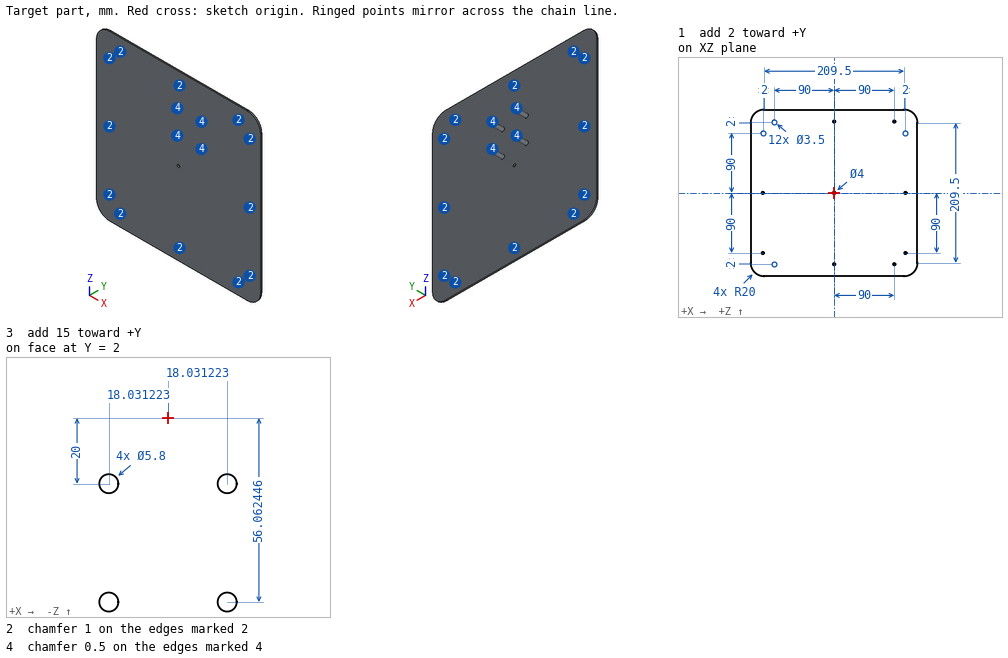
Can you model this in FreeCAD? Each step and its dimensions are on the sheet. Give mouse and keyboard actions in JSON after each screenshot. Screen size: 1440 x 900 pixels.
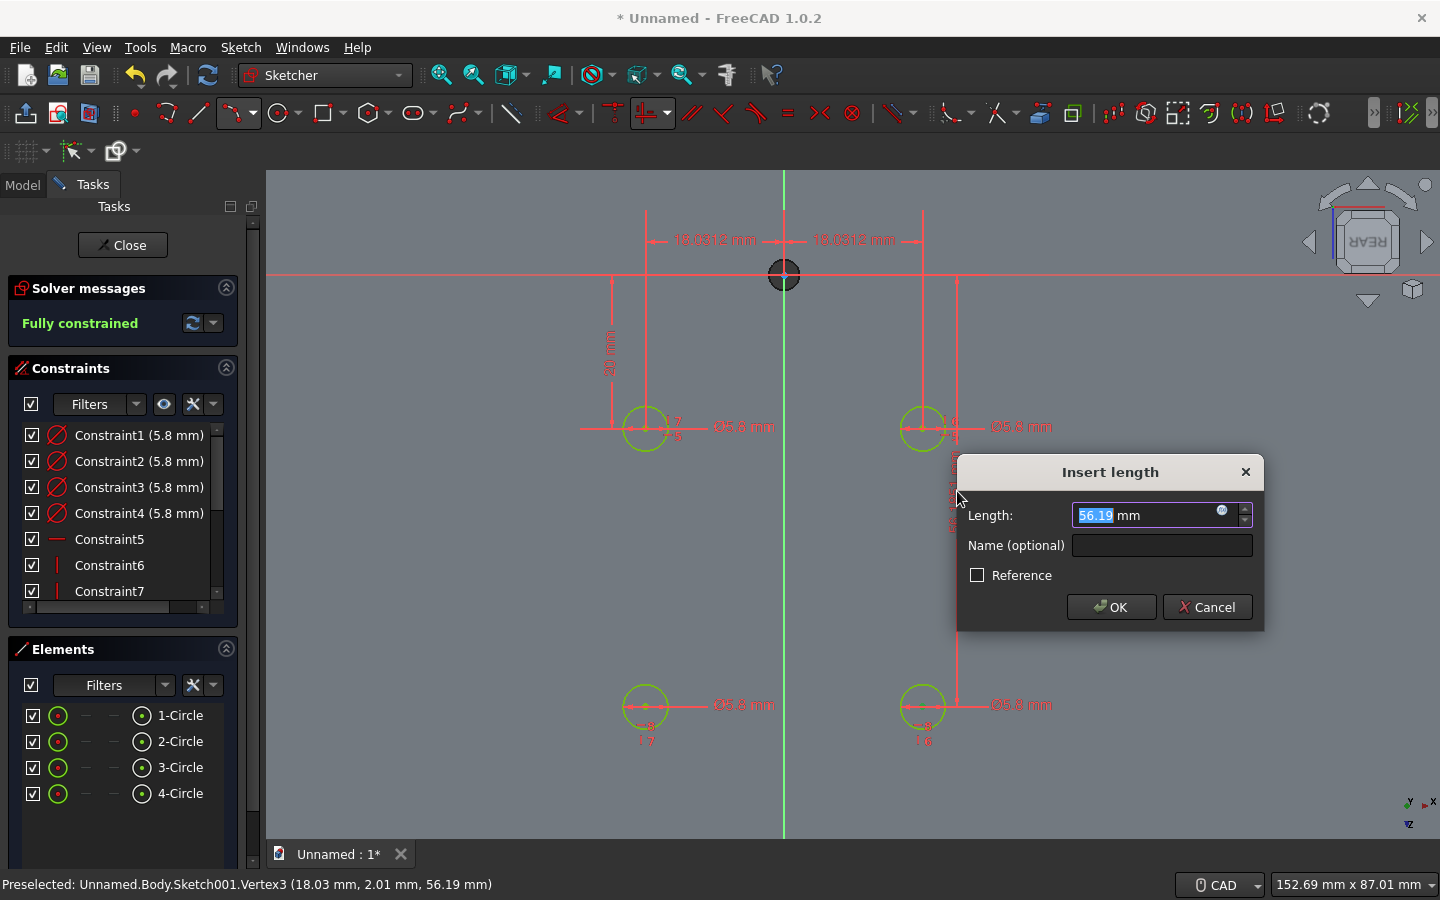
{"action": "type", "text": "56.062446"}
{"action": "key", "text": "Return"}
{"action": "key", "text": "Escape"}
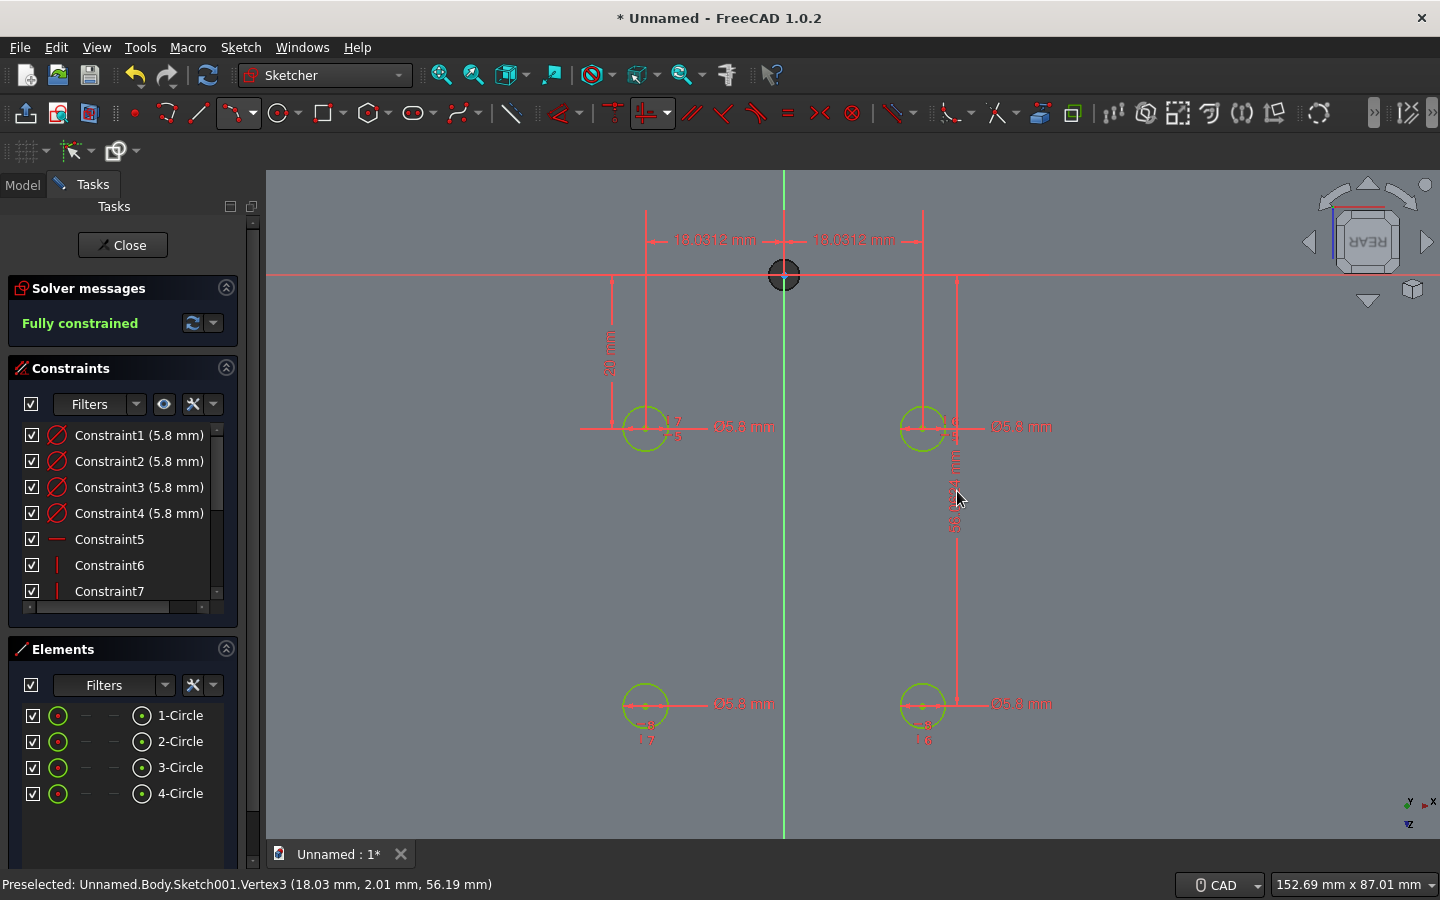
{"action": "left_click", "coordinate": [123, 245]}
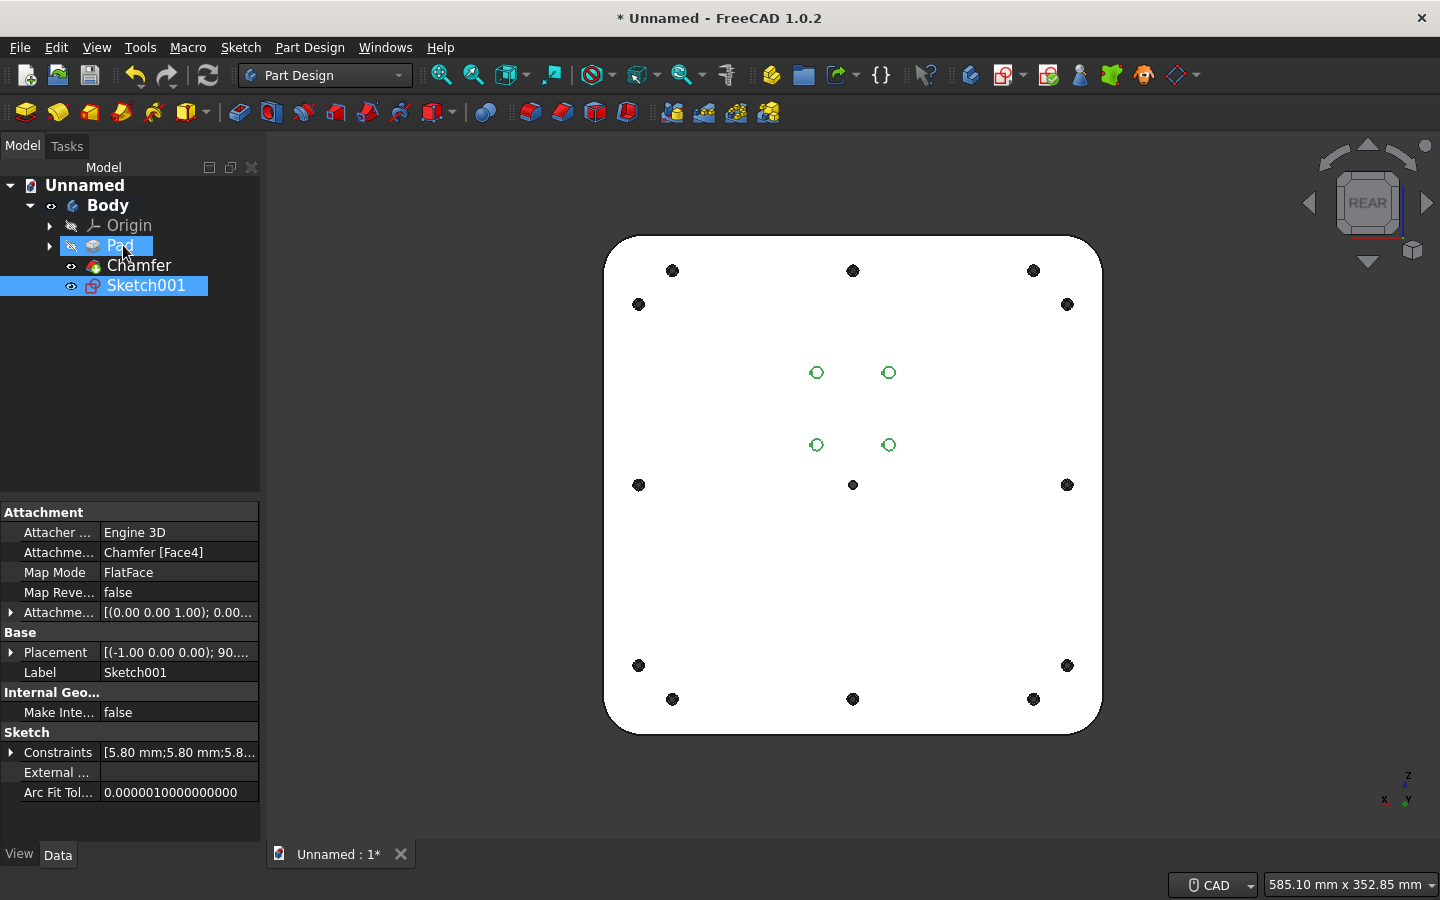
{"action": "left_click", "coordinate": [26, 112]}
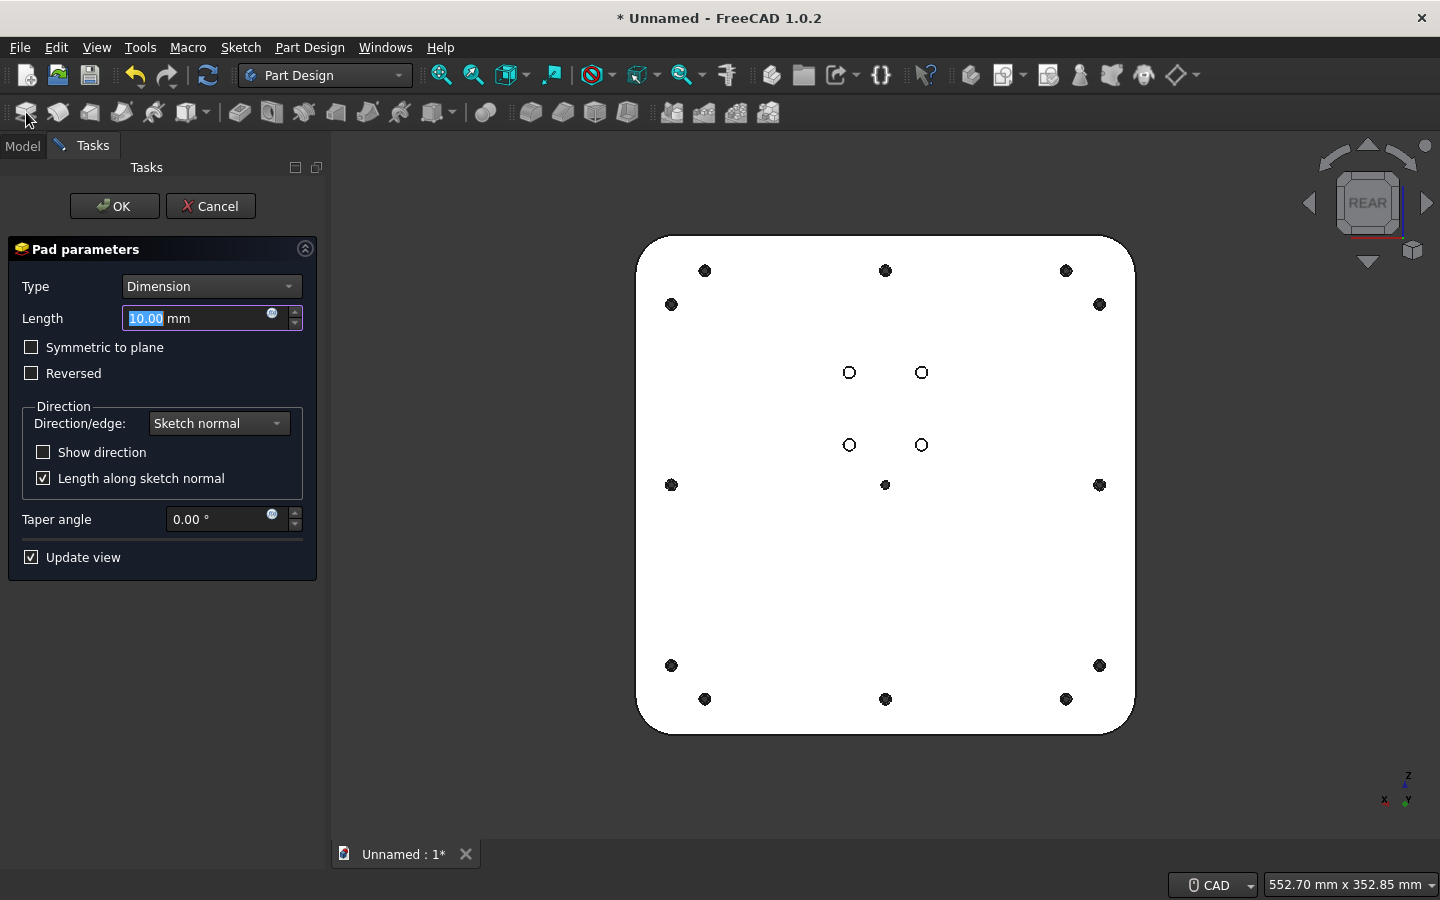
{"action": "type", "text": "15"}
{"action": "key", "text": "Tab"}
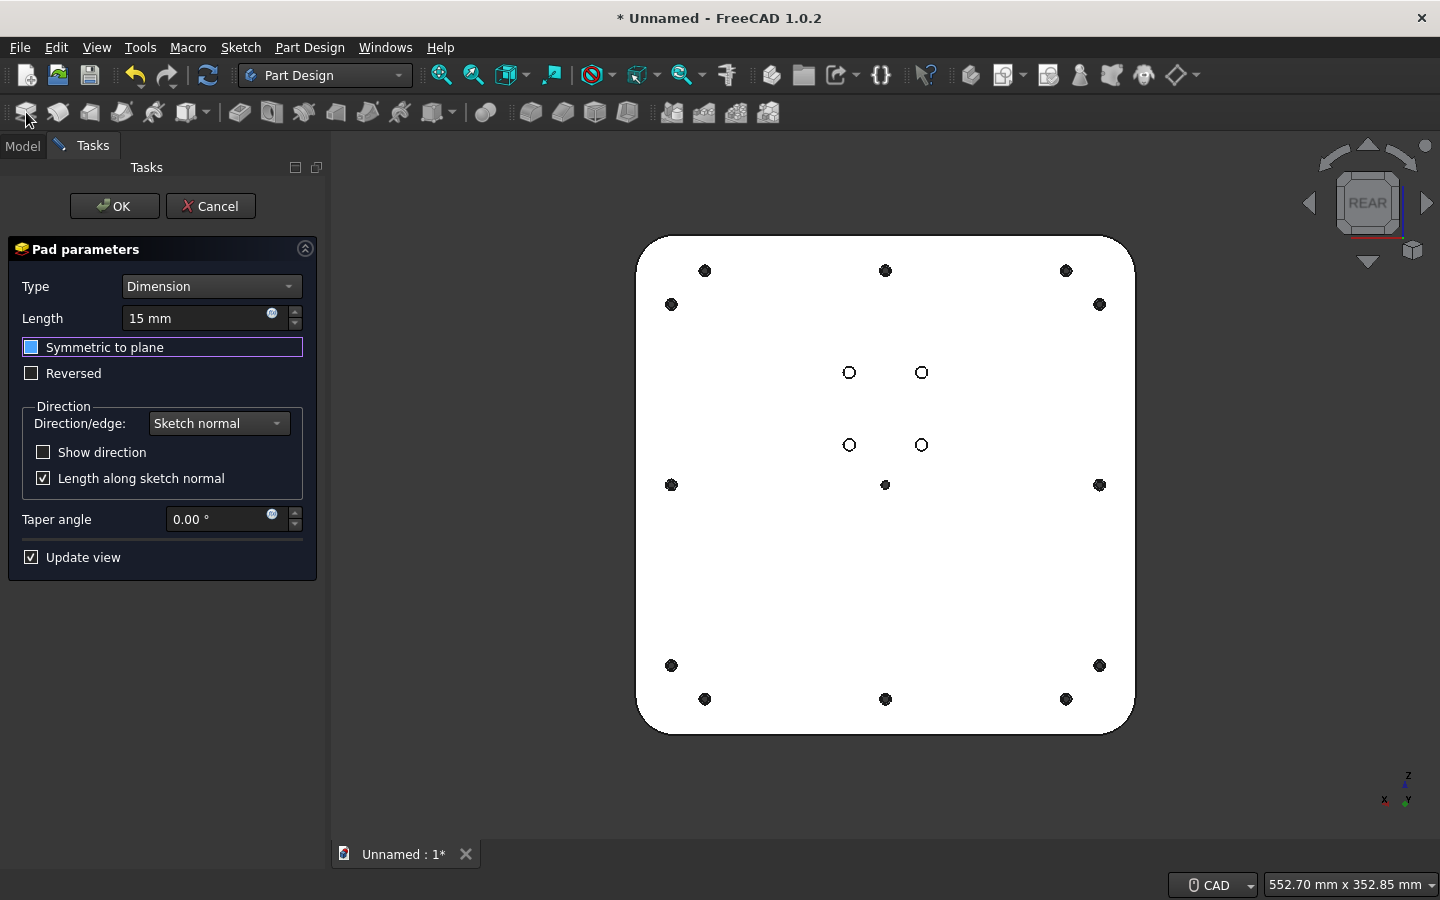
{"action": "left_click", "coordinate": [115, 206]}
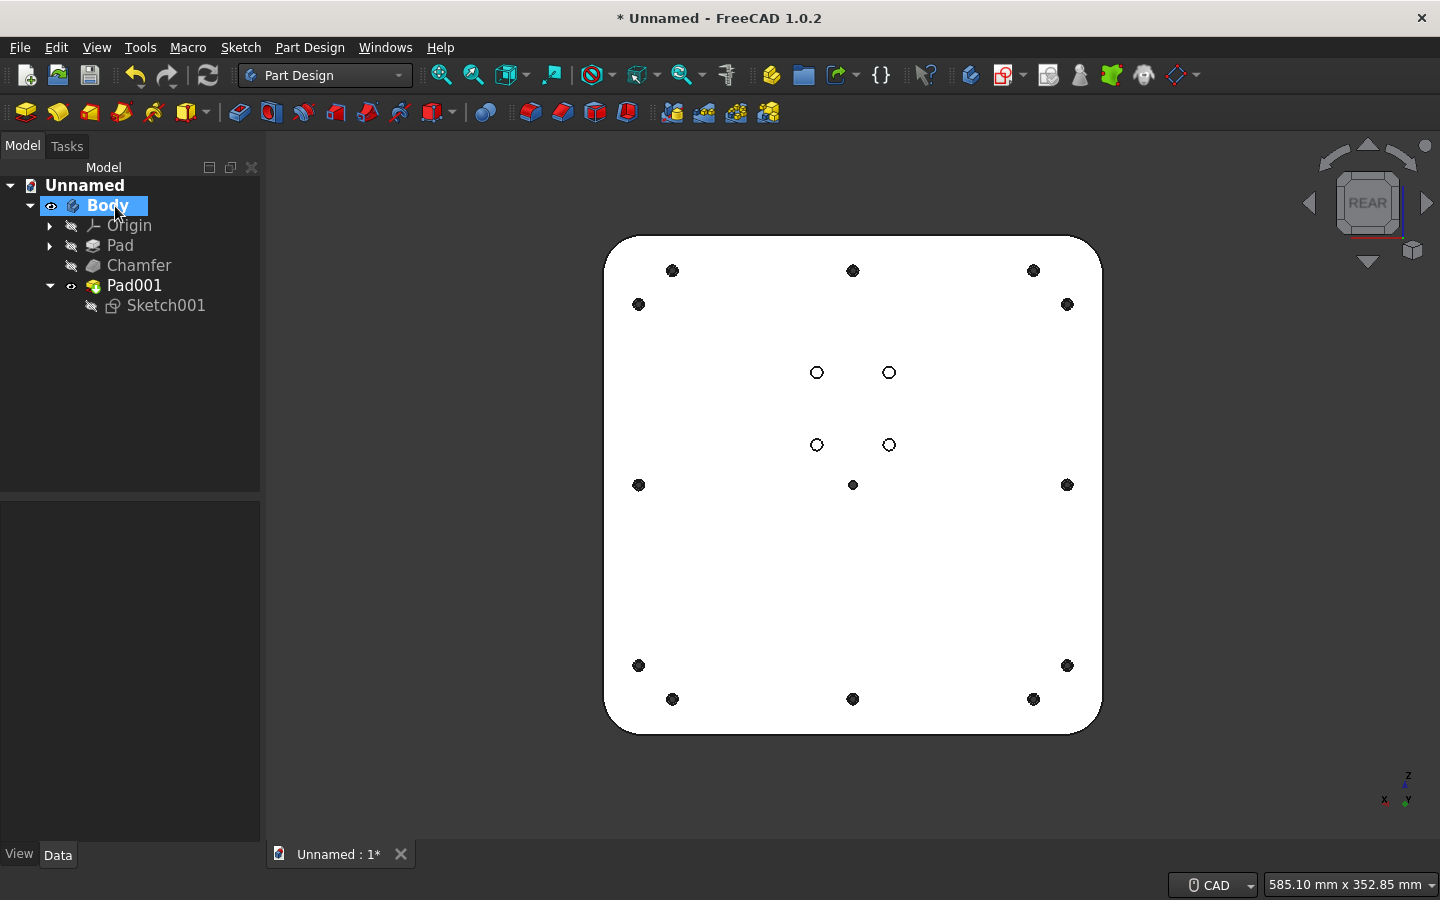
{"action": "left_click", "coordinate": [895, 444]}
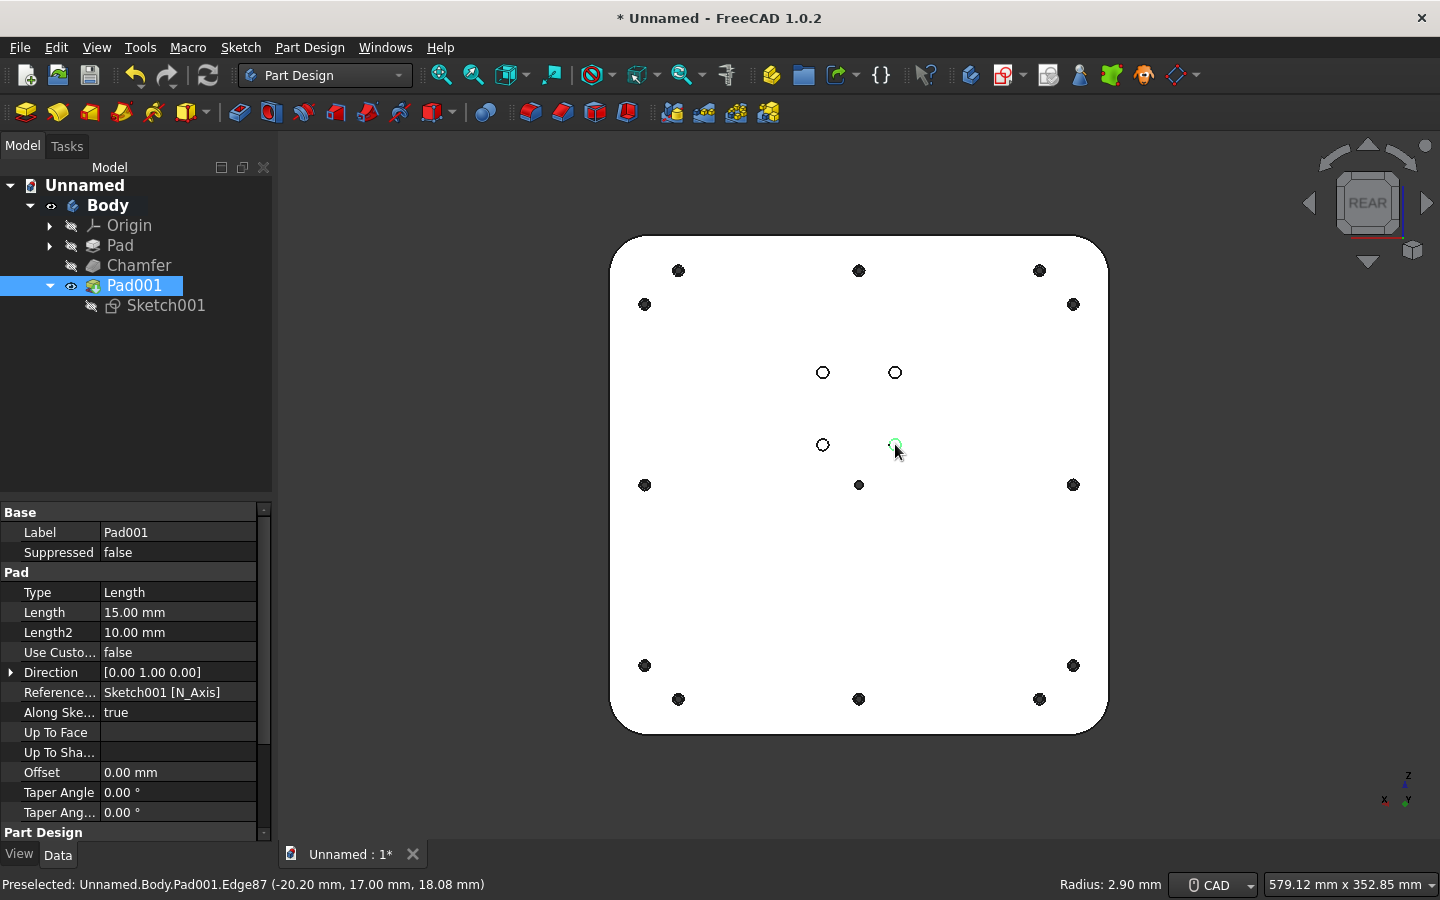
{"action": "left_click", "coordinate": [829, 444], "text": "ctrl"}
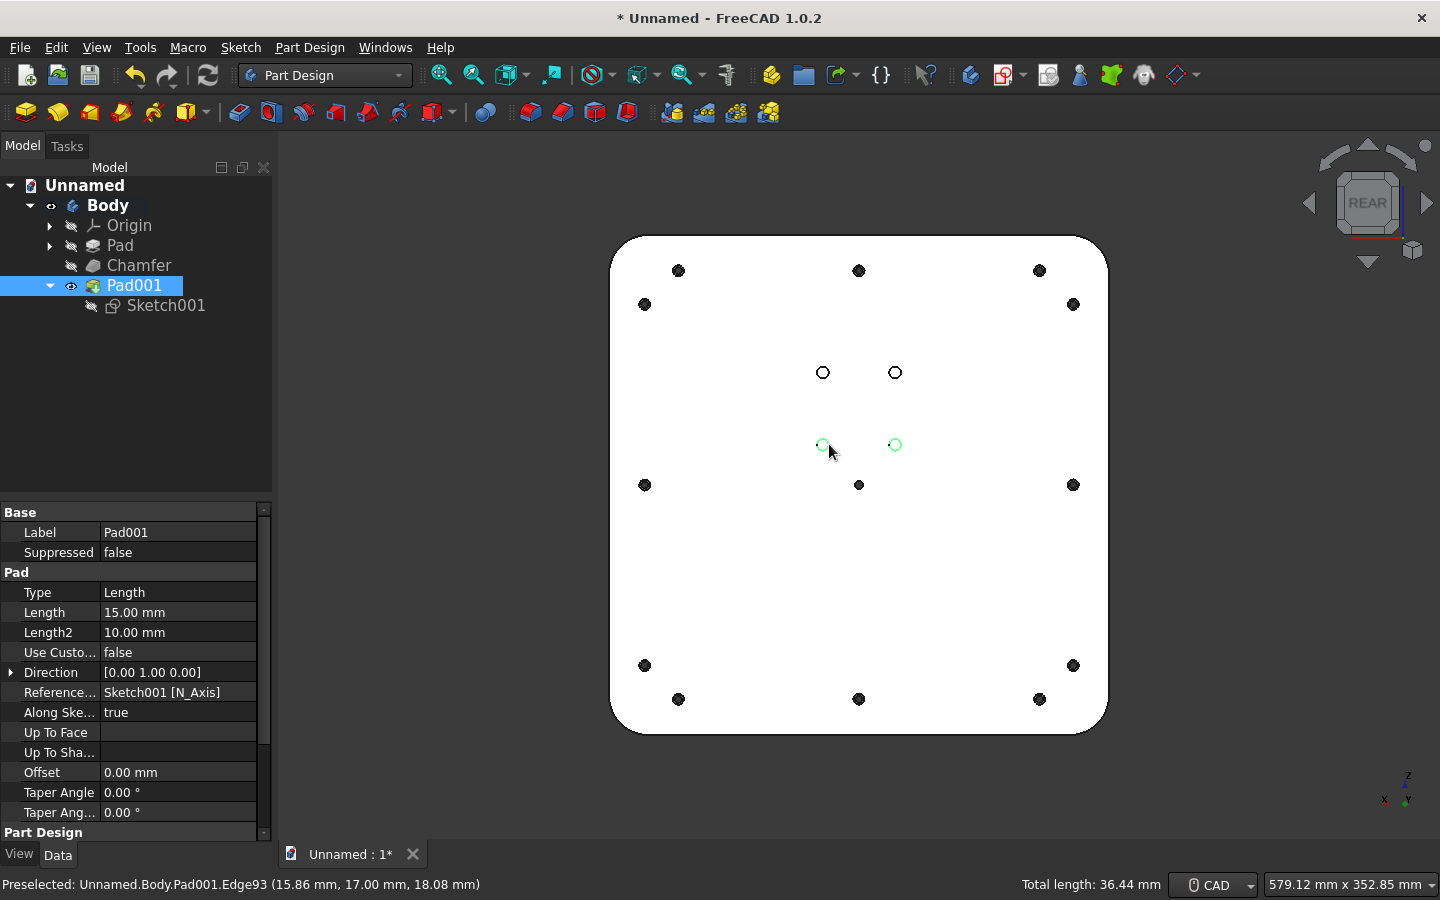
{"action": "left_click", "coordinate": [829, 372], "text": "ctrl"}